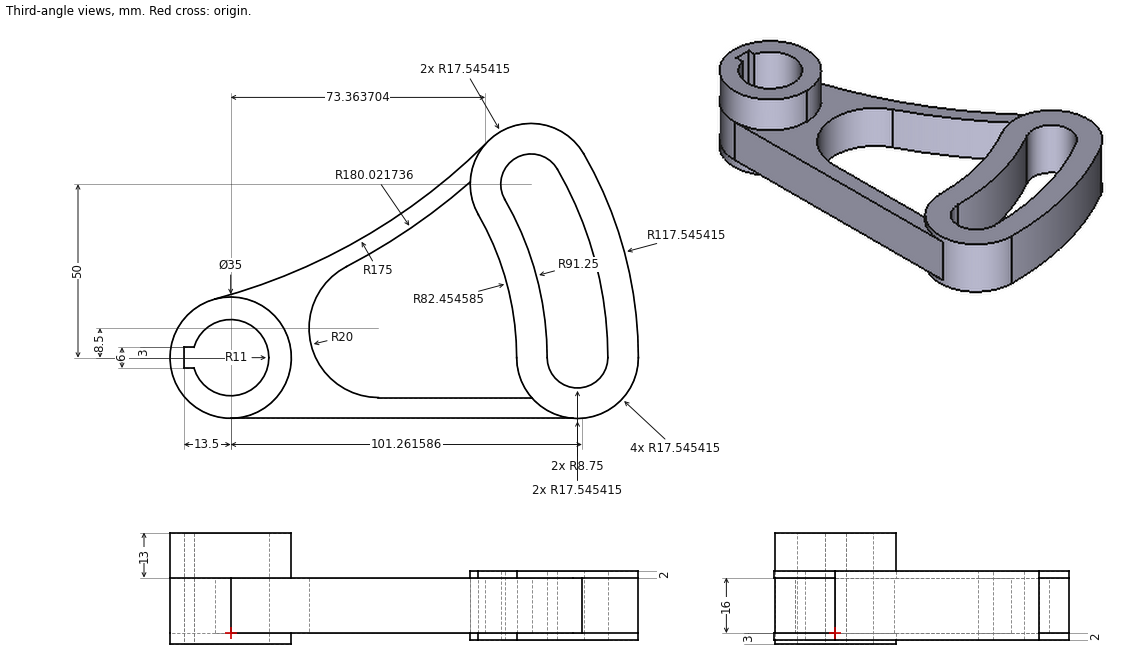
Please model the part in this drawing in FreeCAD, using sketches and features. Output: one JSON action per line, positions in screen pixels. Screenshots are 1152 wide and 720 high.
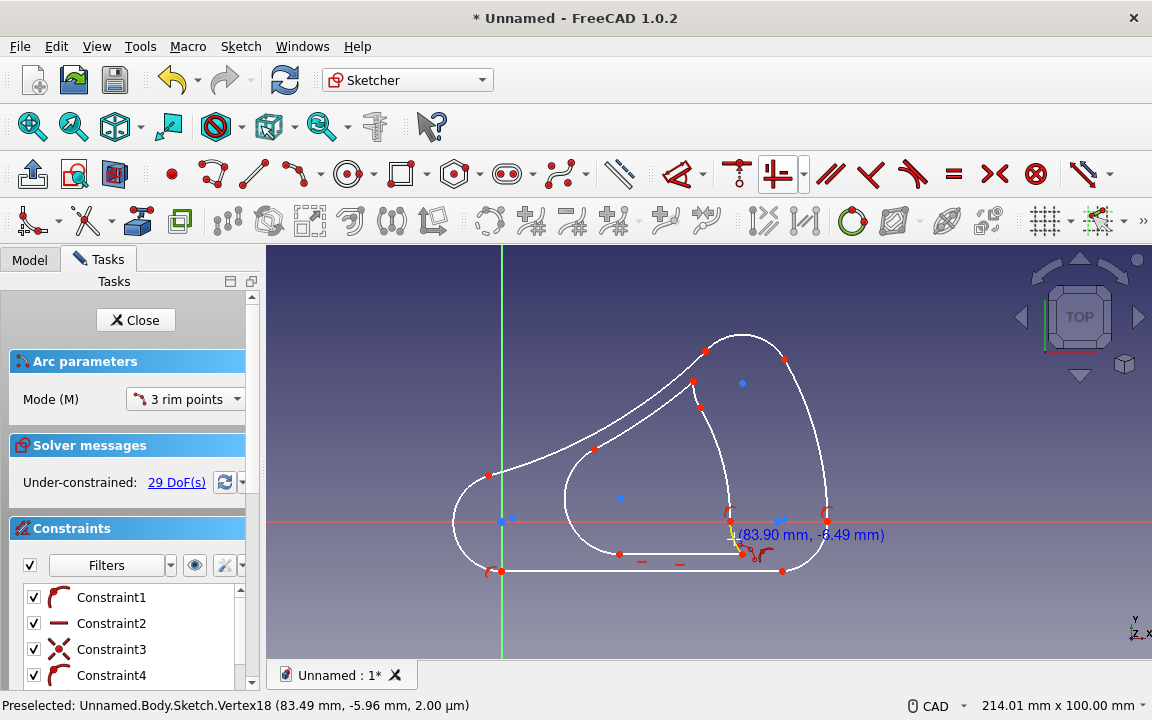
{"action": "left_click", "coordinate": [721, 395]}
{"action": "left_click", "coordinate": [763, 371]}
{"action": "left_click", "coordinate": [730, 362]}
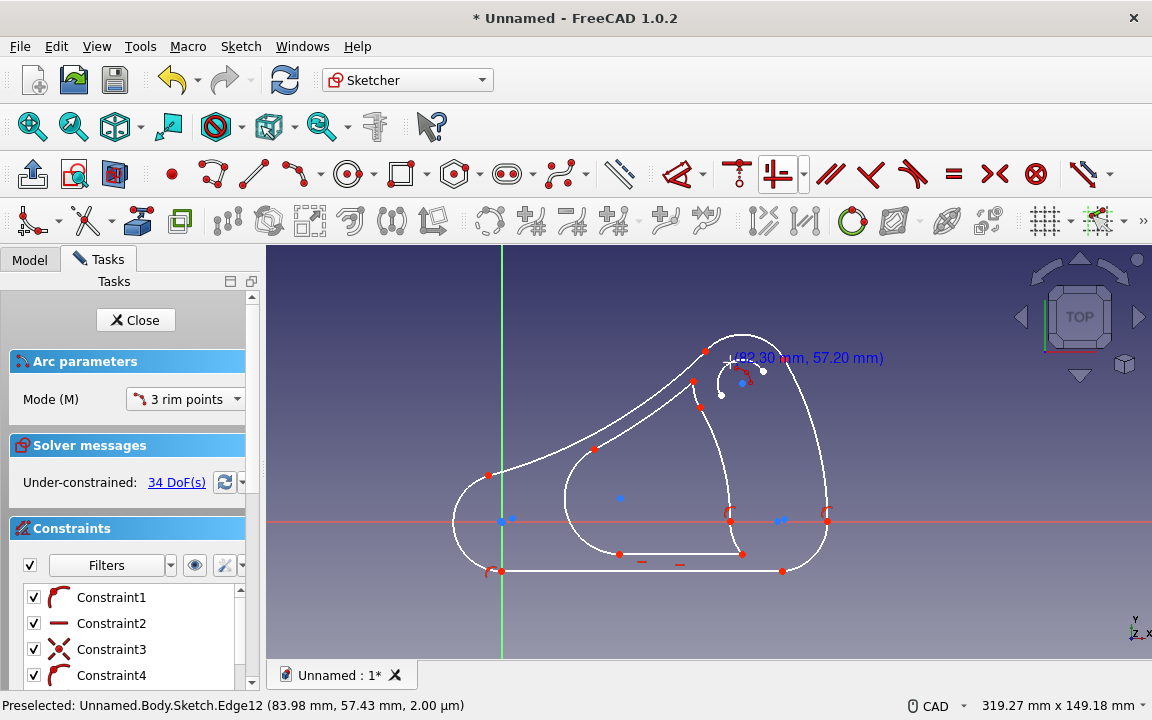
{"action": "left_click", "coordinate": [763, 372]}
{"action": "left_click", "coordinate": [803, 522]}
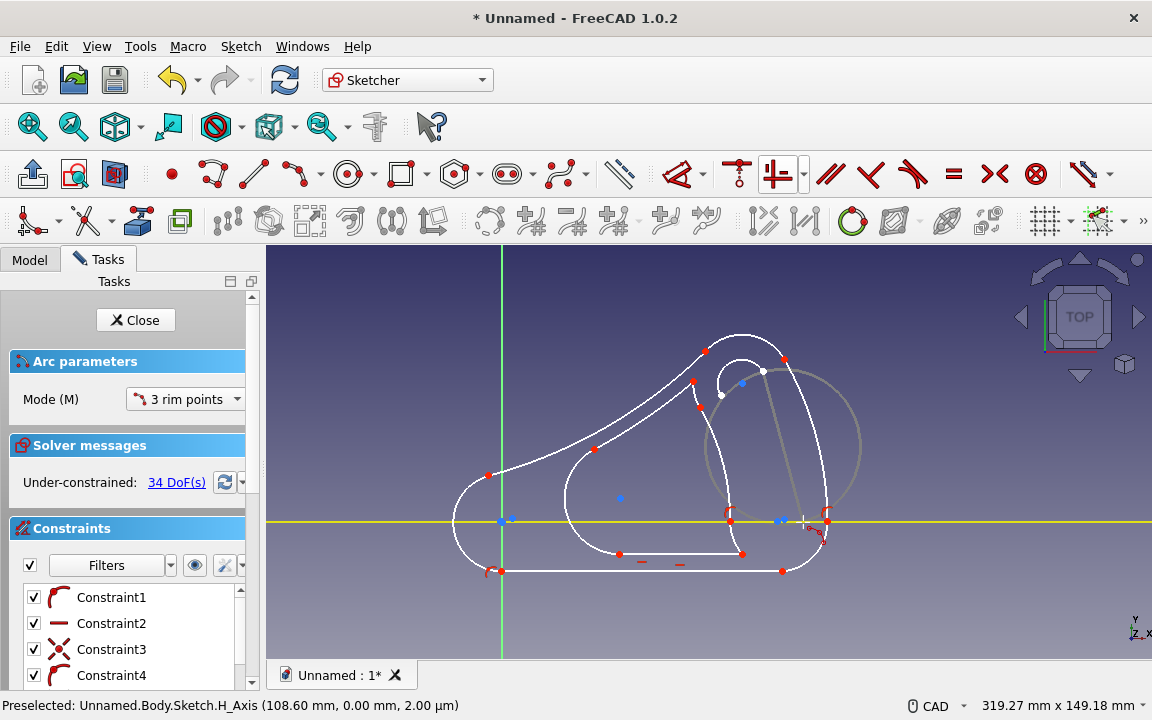
{"action": "scroll", "coordinate": [793, 444], "scroll_direction": "up", "scroll_amount": 3}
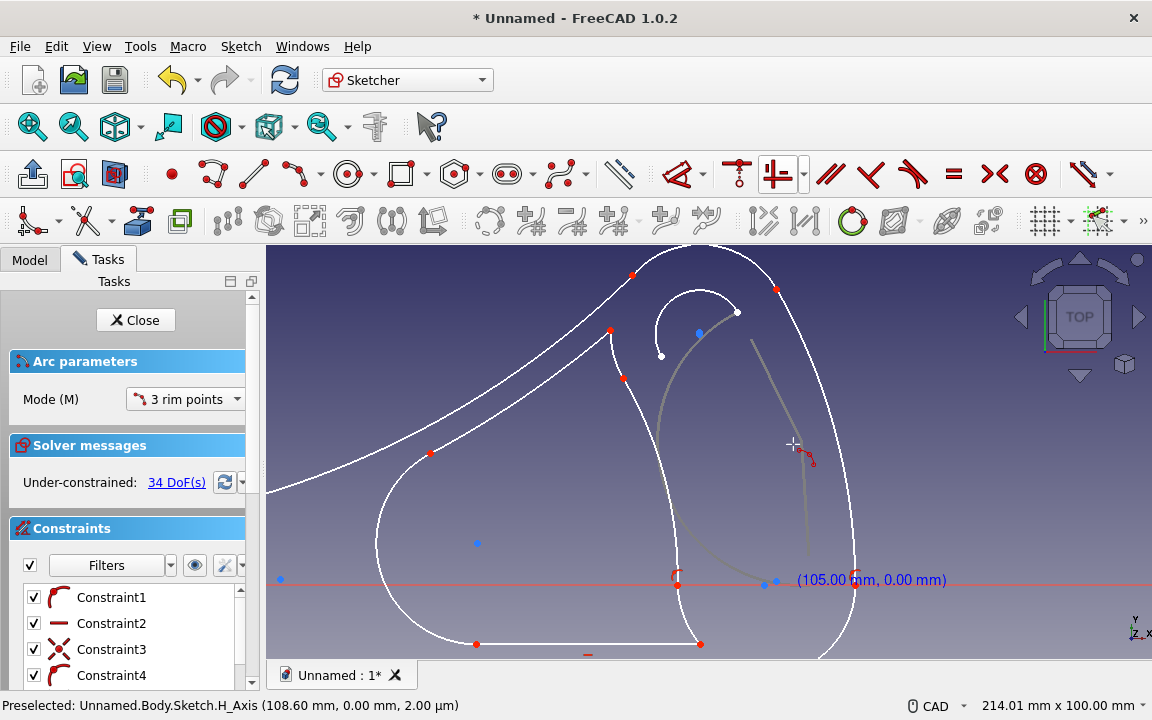
{"action": "left_click", "coordinate": [793, 443]}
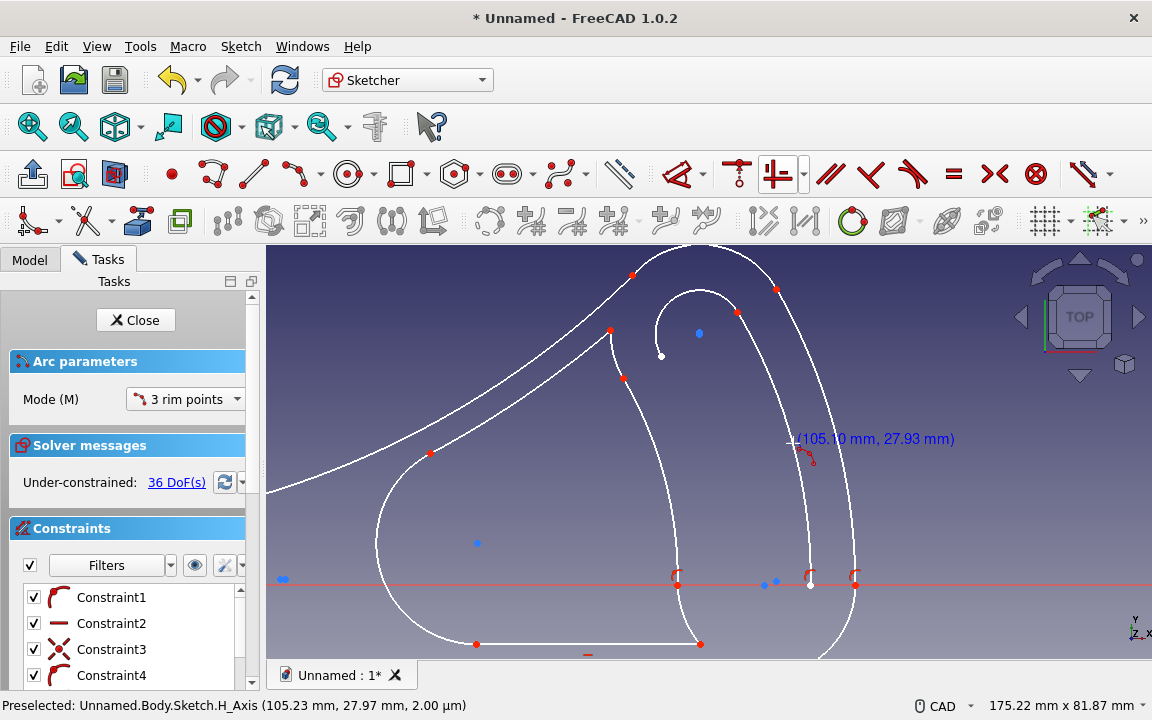
{"action": "left_click", "coordinate": [811, 585]}
{"action": "left_click", "coordinate": [723, 585]}
{"action": "left_click", "coordinate": [767, 629]}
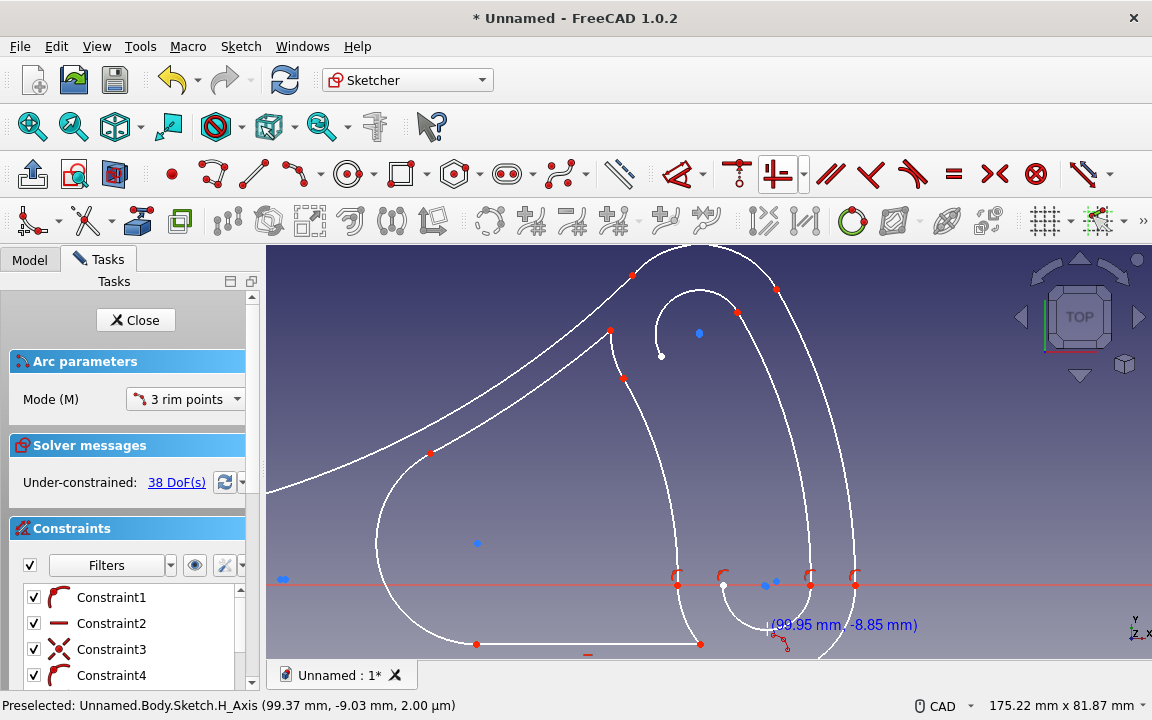
{"action": "left_click", "coordinate": [723, 585]}
{"action": "left_click", "coordinate": [661, 356]}
{"action": "left_click", "coordinate": [707, 466]}
{"action": "key", "text": "Escape"}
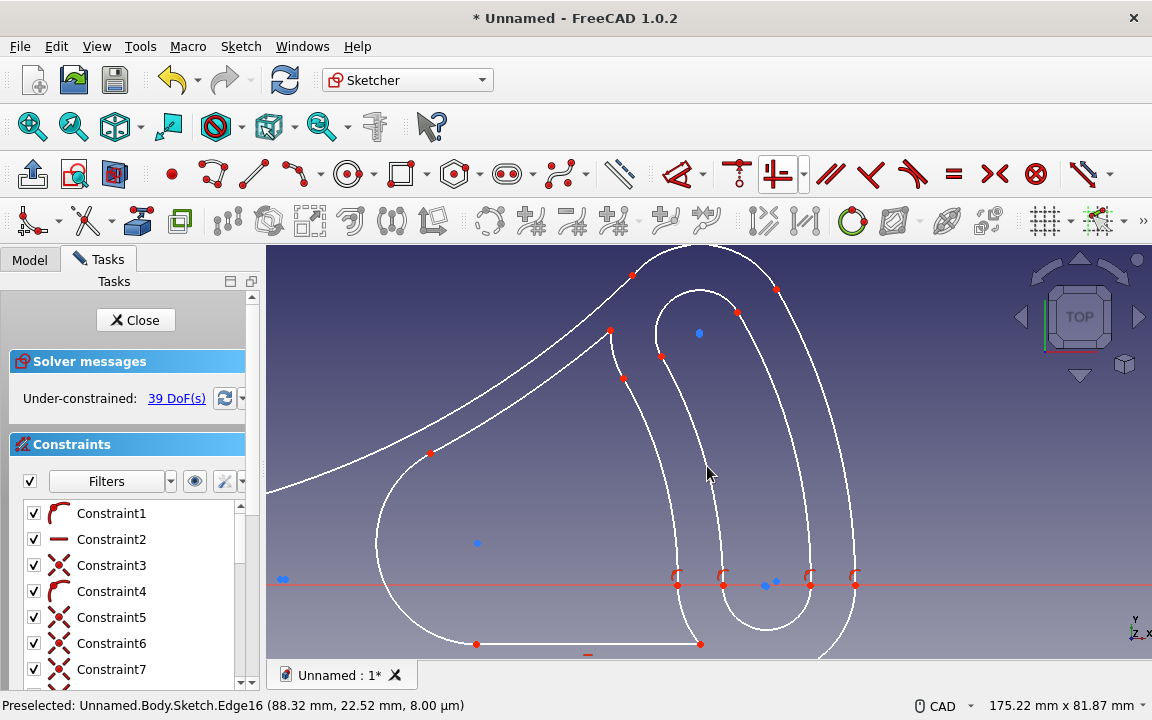
{"action": "scroll", "coordinate": [793, 444], "scroll_direction": "down", "scroll_amount": 3}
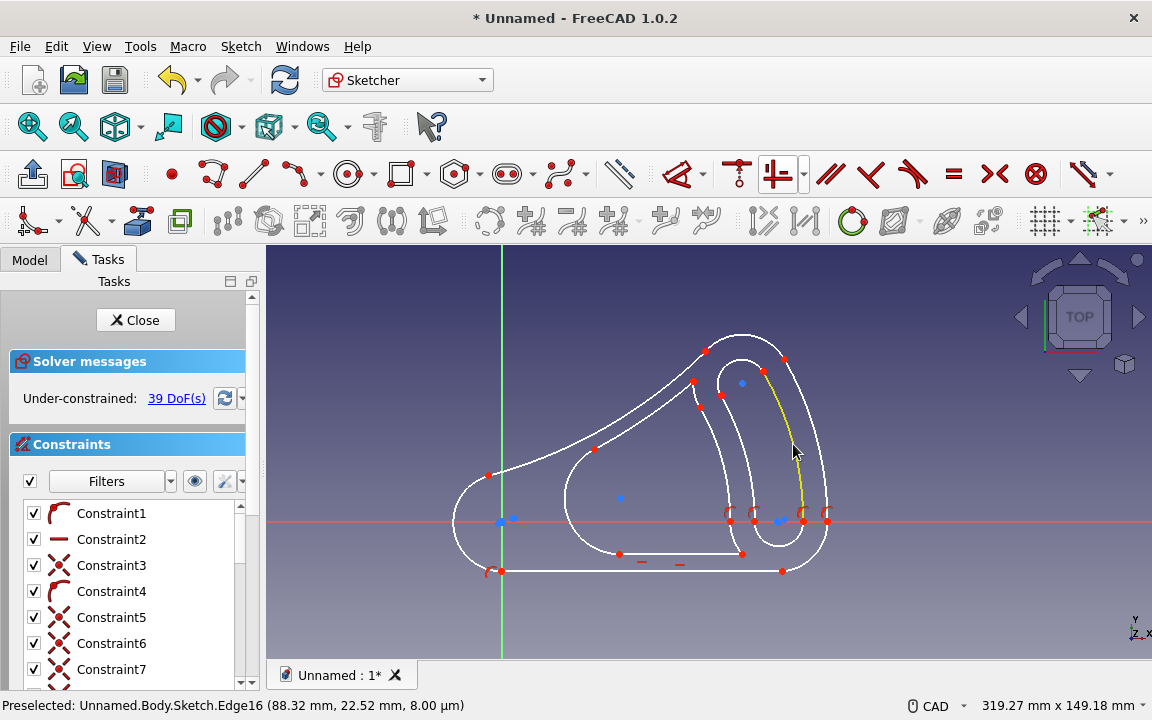
{"action": "left_click", "coordinate": [586, 571]}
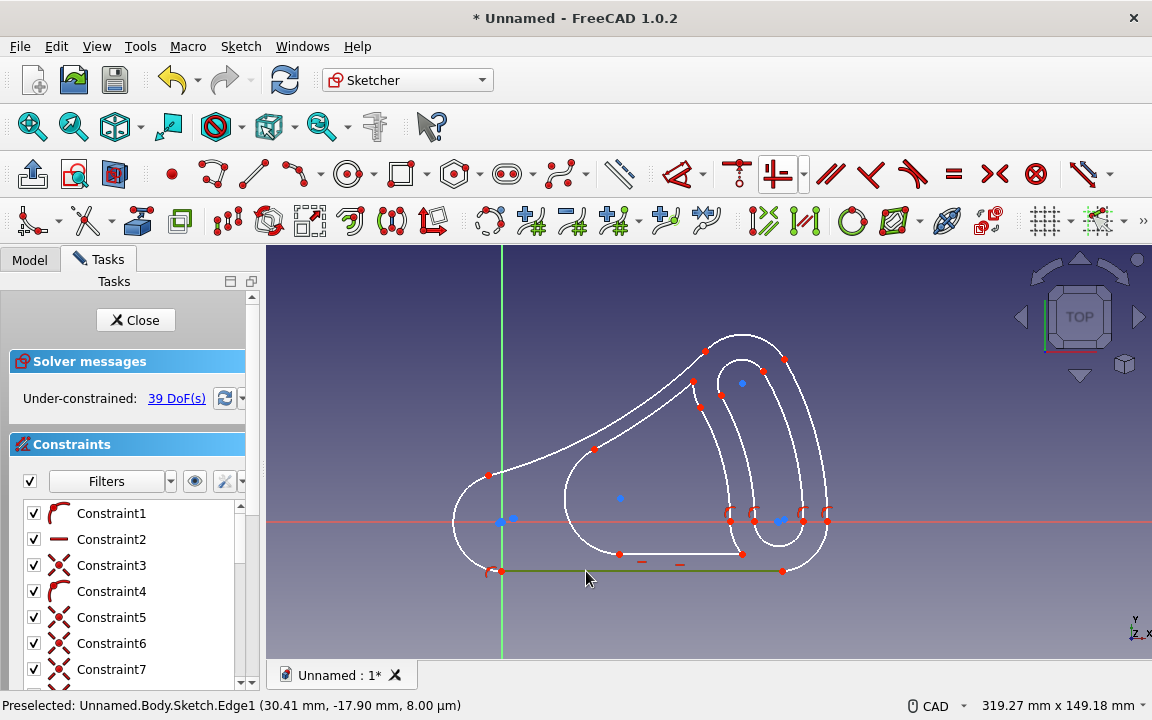
{"action": "left_click", "coordinate": [458, 502]}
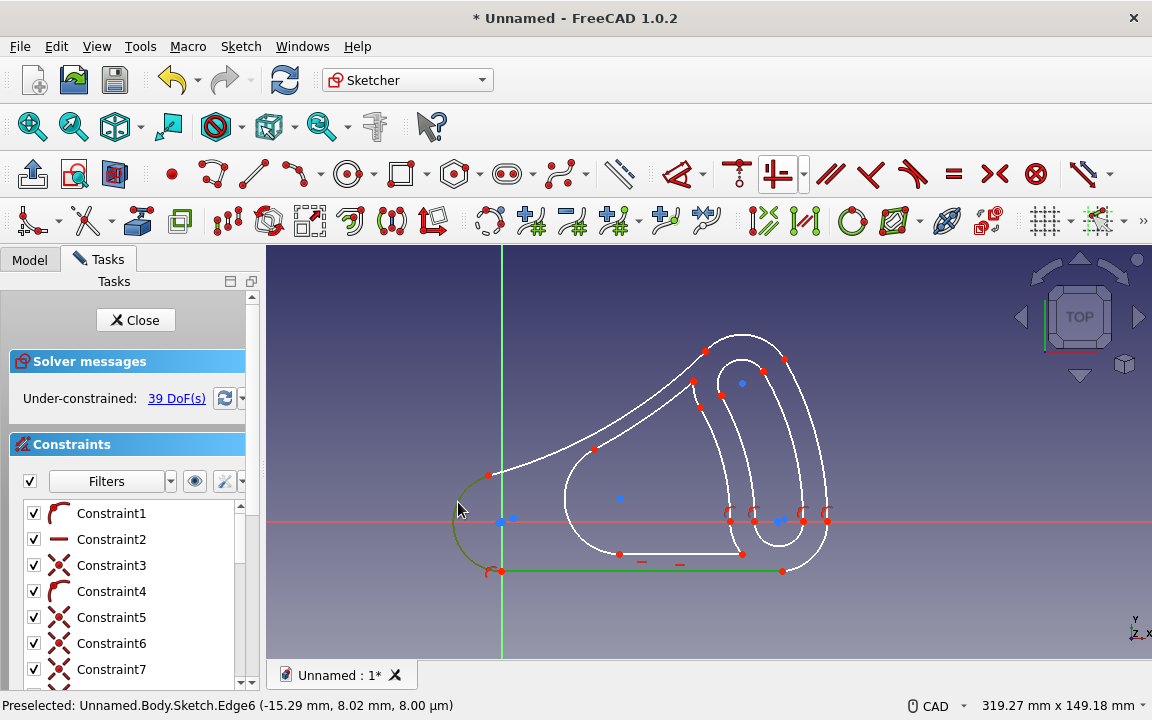
{"action": "left_click", "coordinate": [913, 174]}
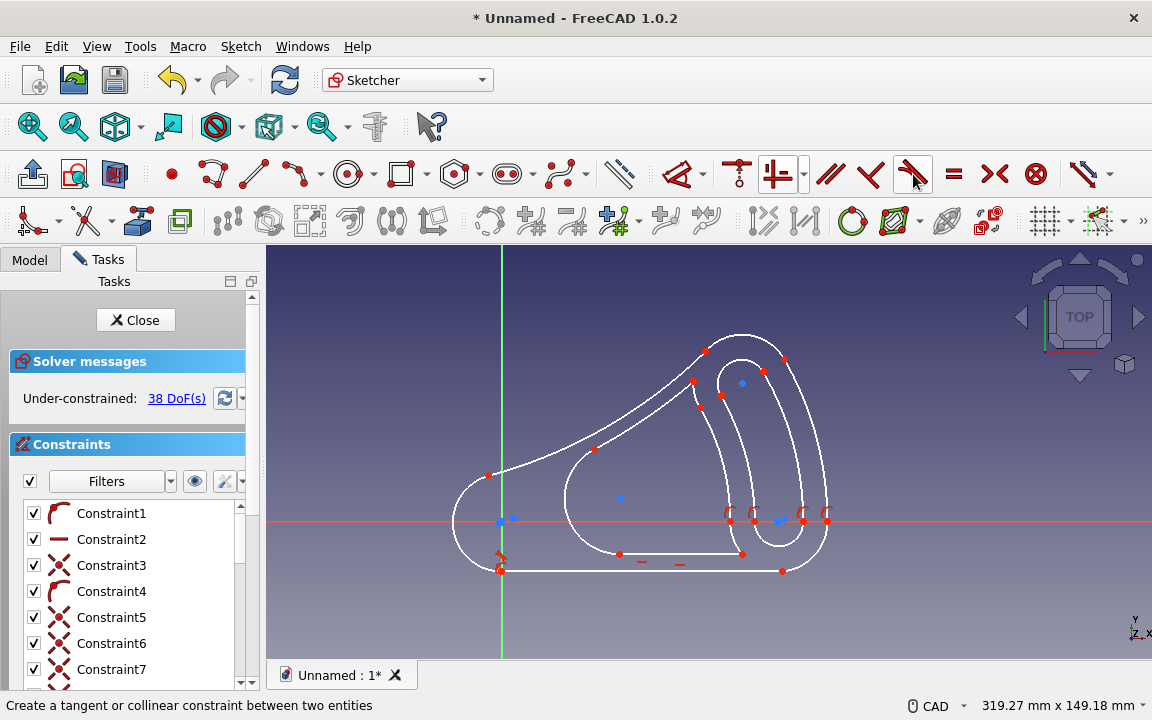
{"action": "left_click", "coordinate": [803, 565]}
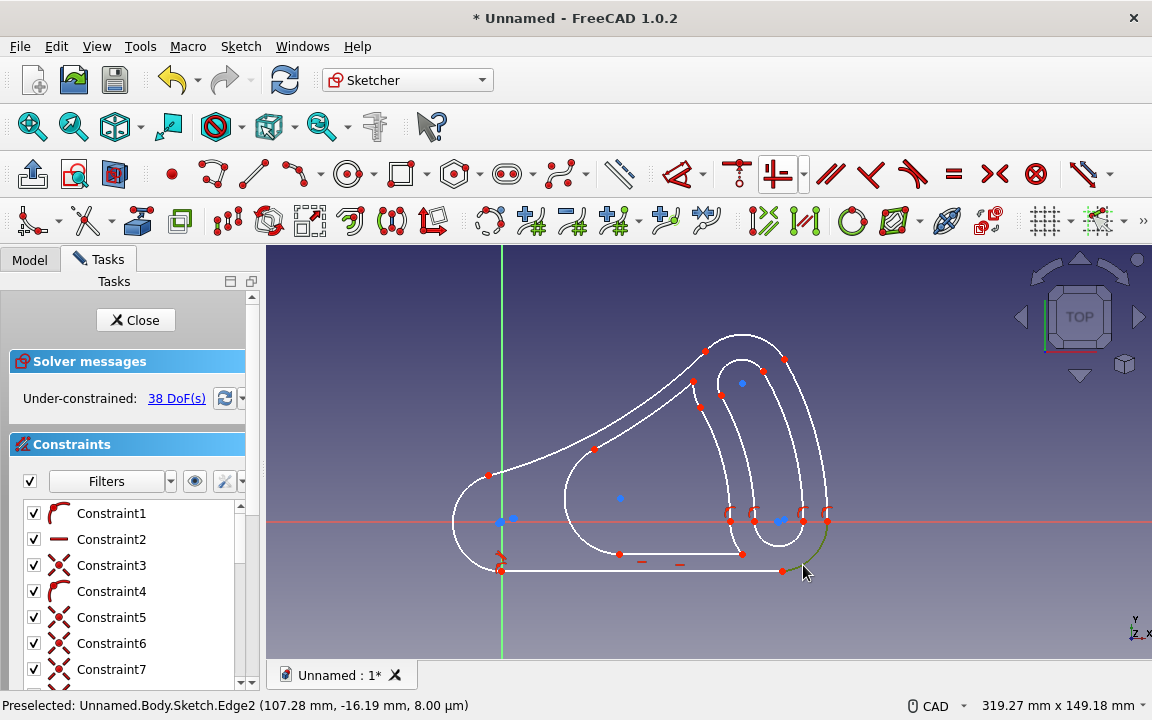
{"action": "left_click", "coordinate": [824, 471]}